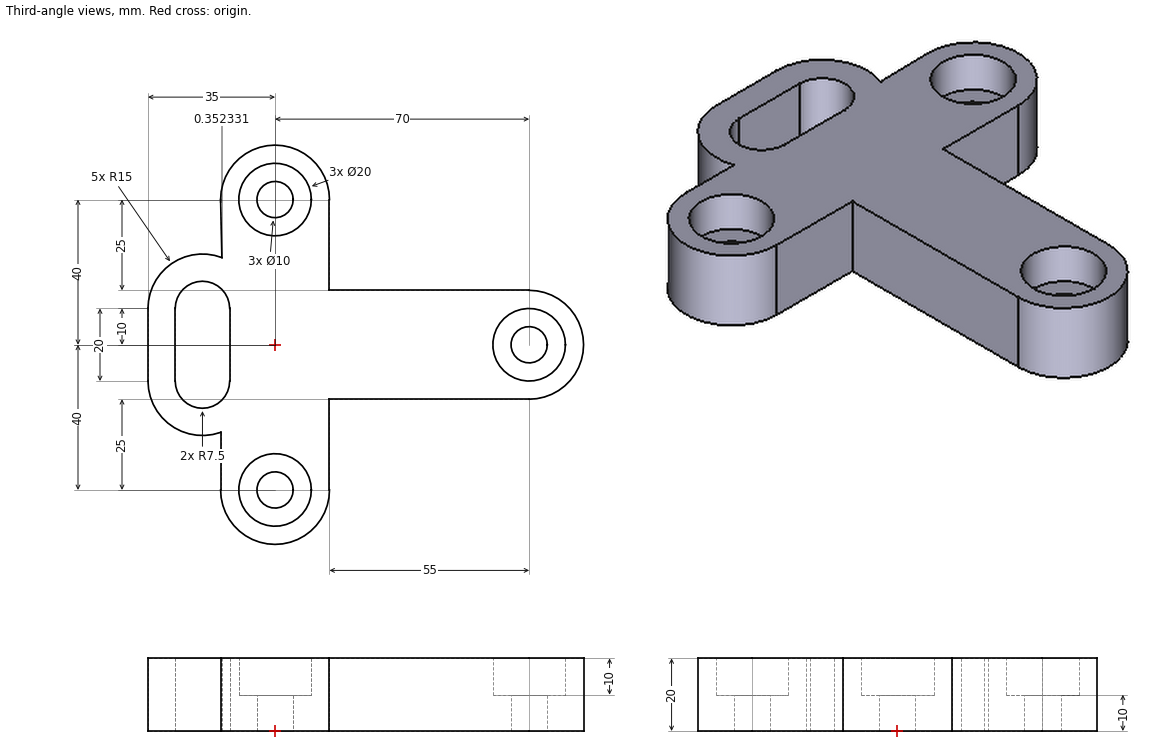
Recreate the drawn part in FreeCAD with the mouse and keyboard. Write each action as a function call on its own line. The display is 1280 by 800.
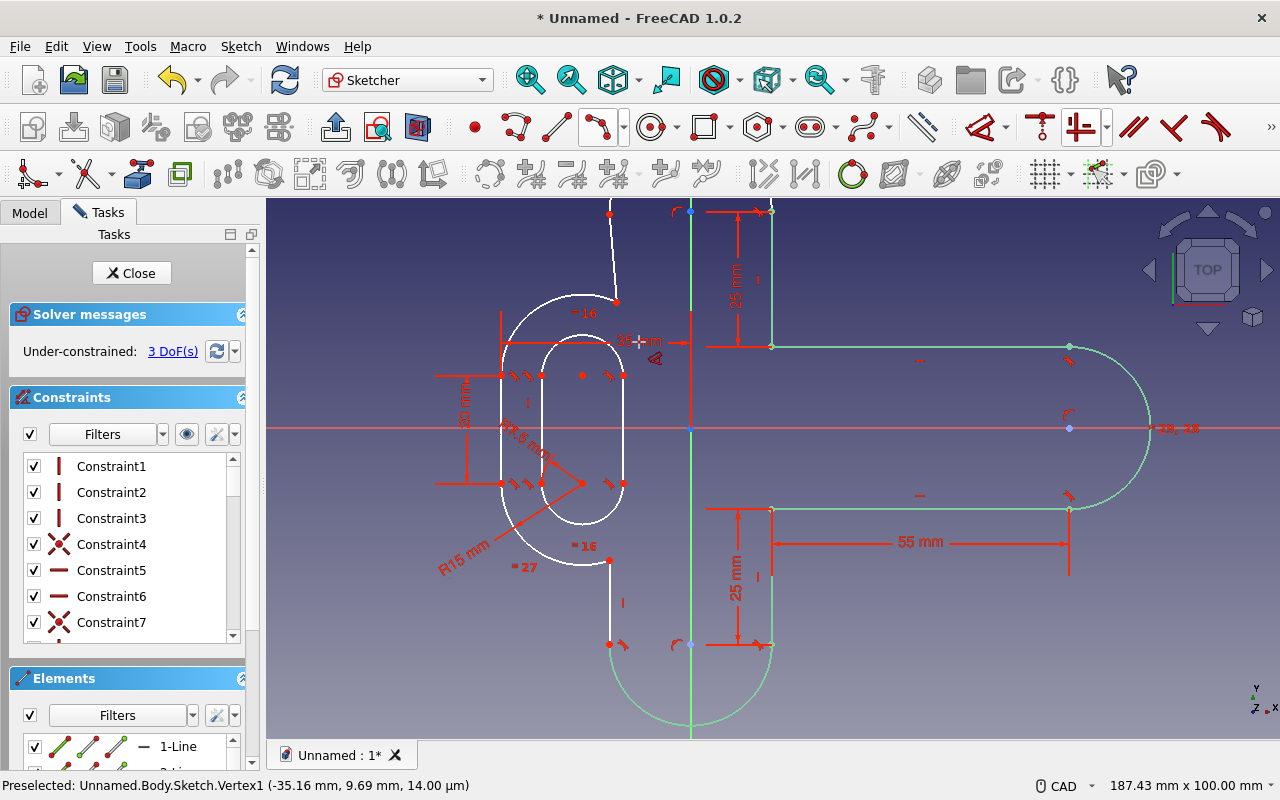
click(501, 376)
click(467, 384)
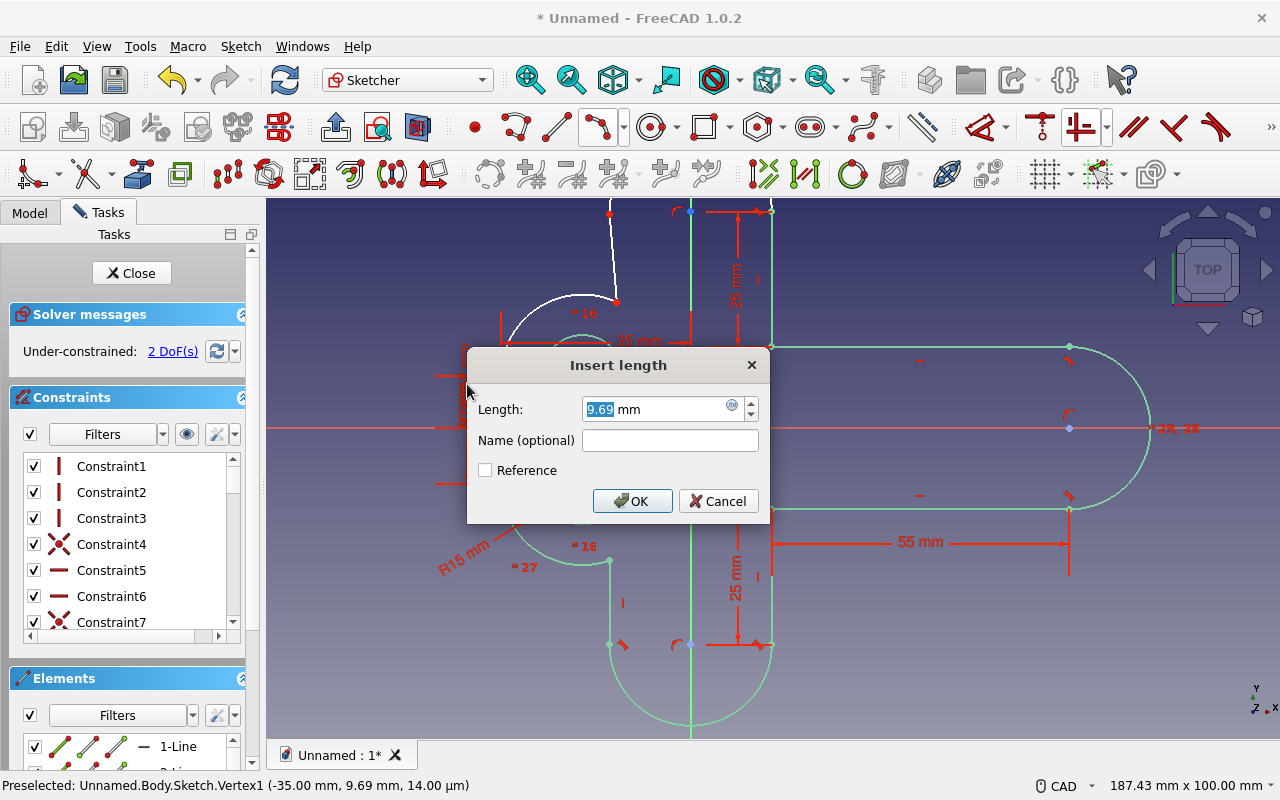
text(10)
key(Return)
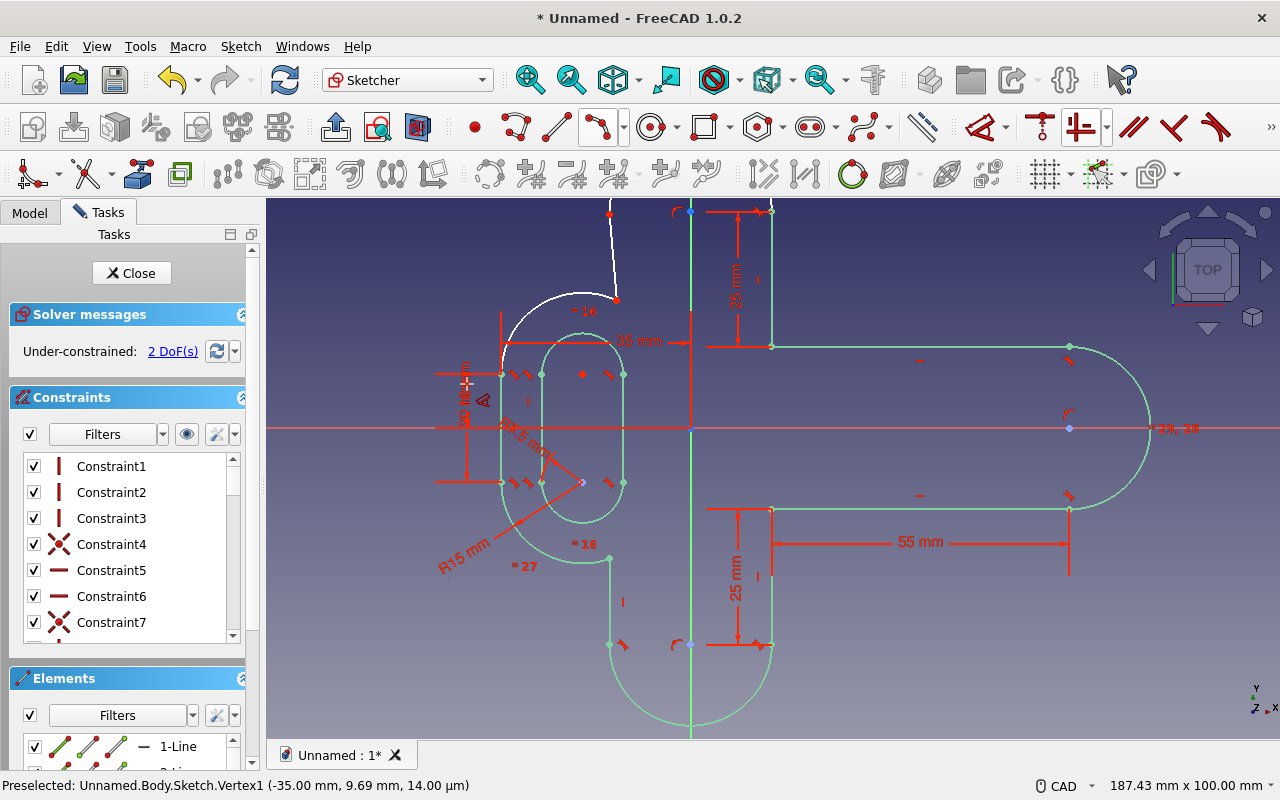
scroll(557, 518, down, 3)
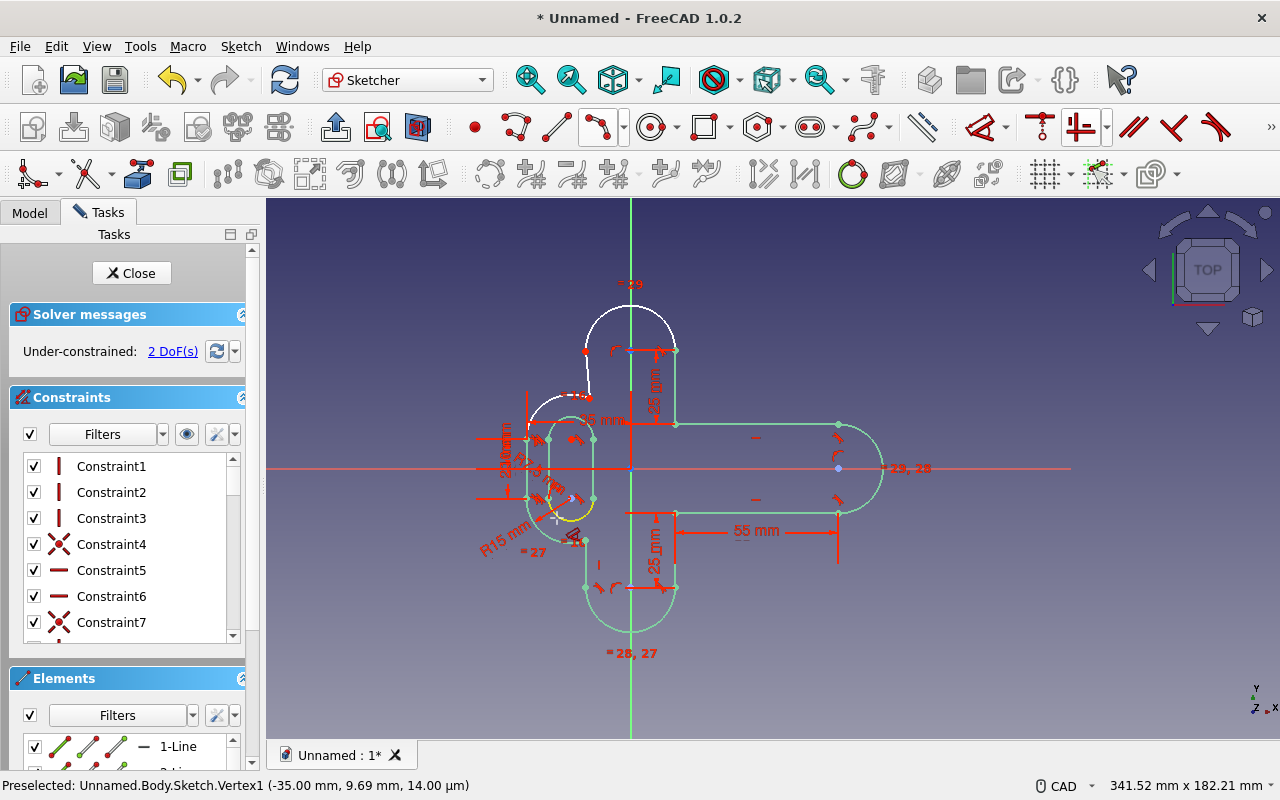
click(586, 351)
click(552, 383)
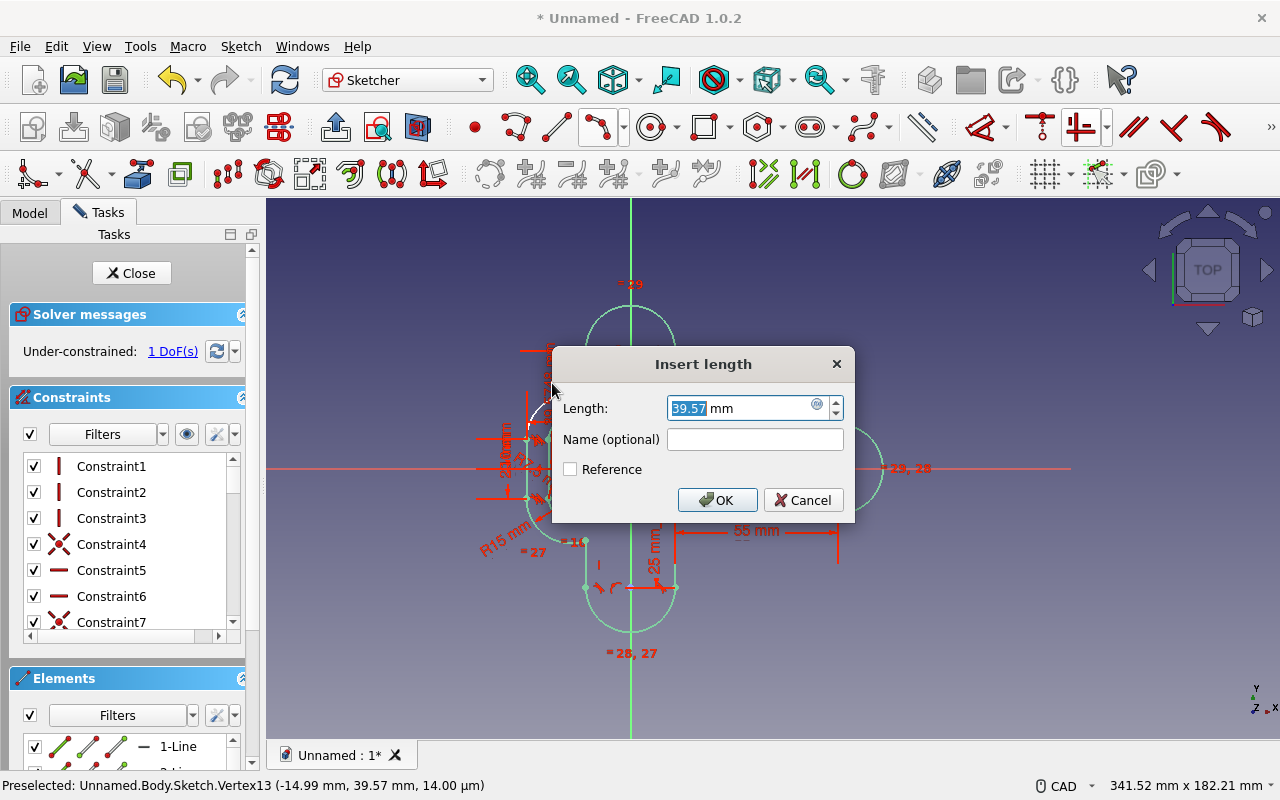
text(40)
key(Return)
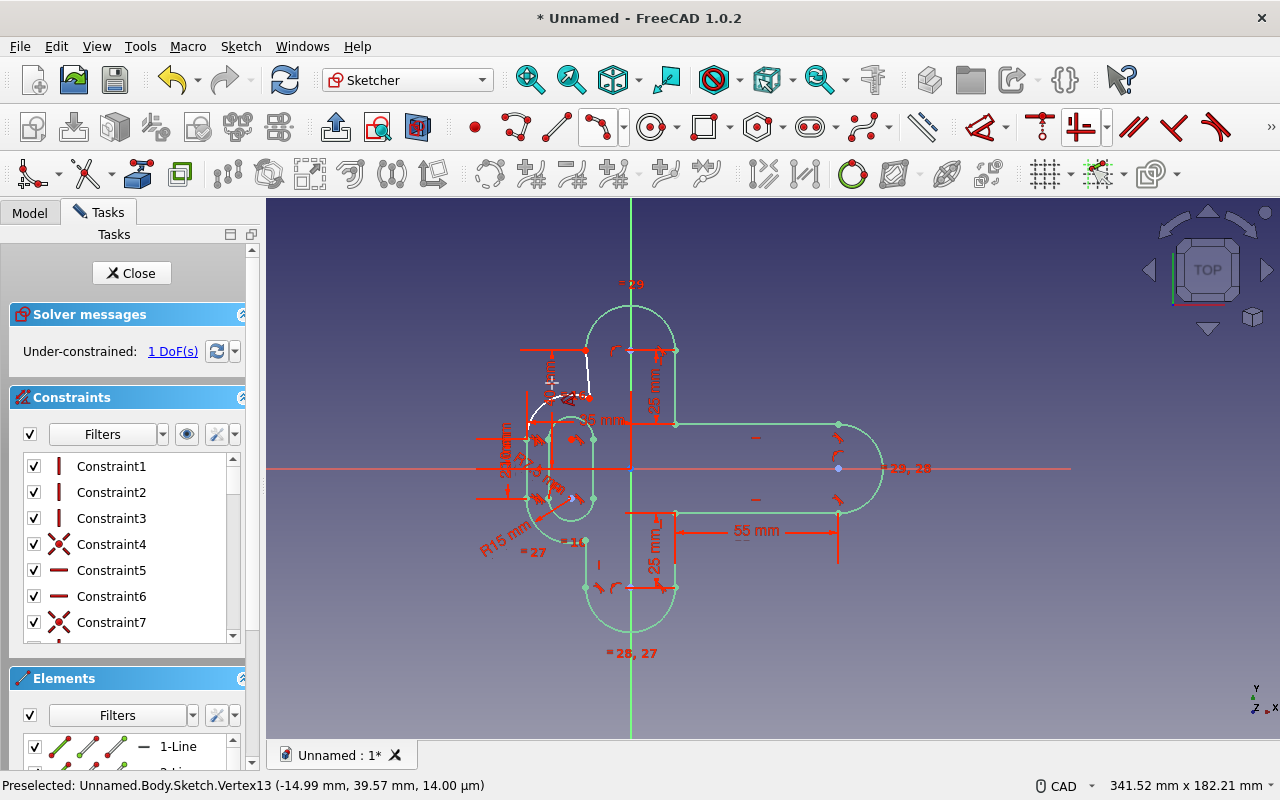
scroll(587, 365, up, 19)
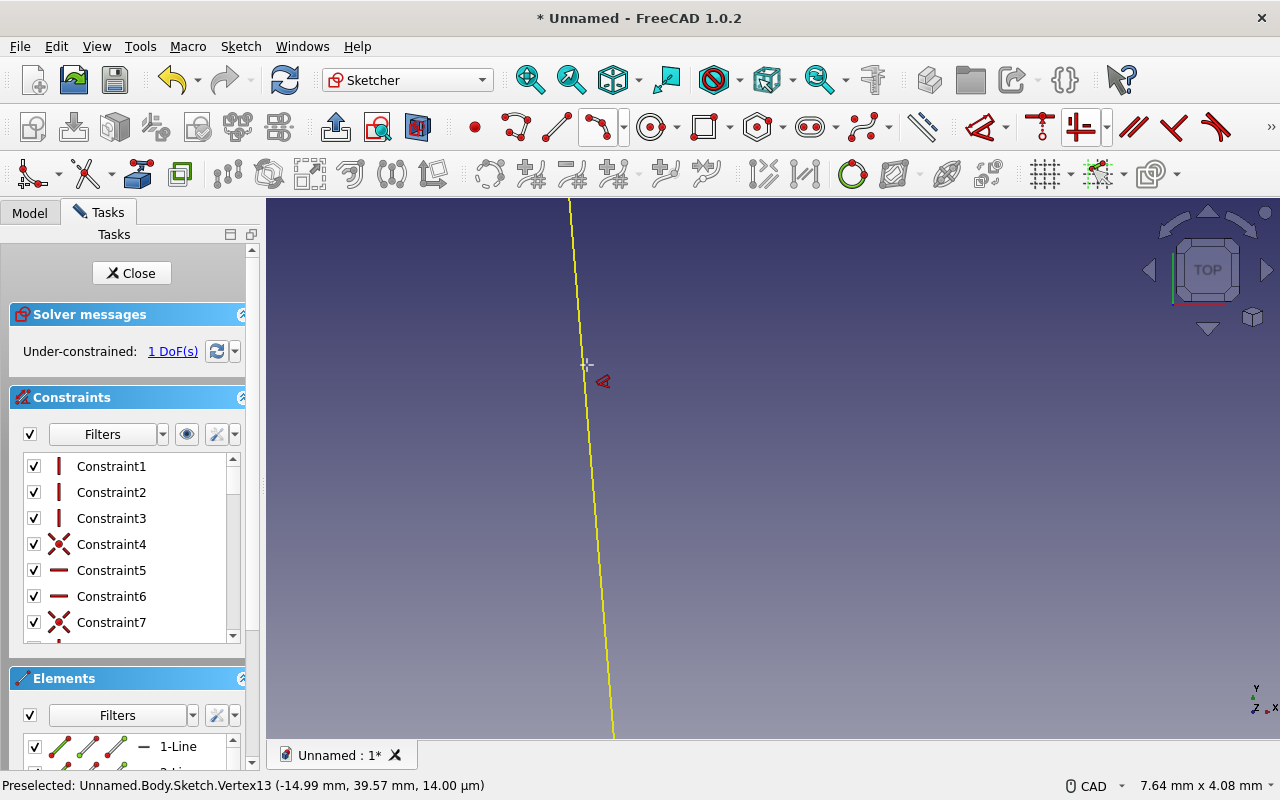
click(581, 343)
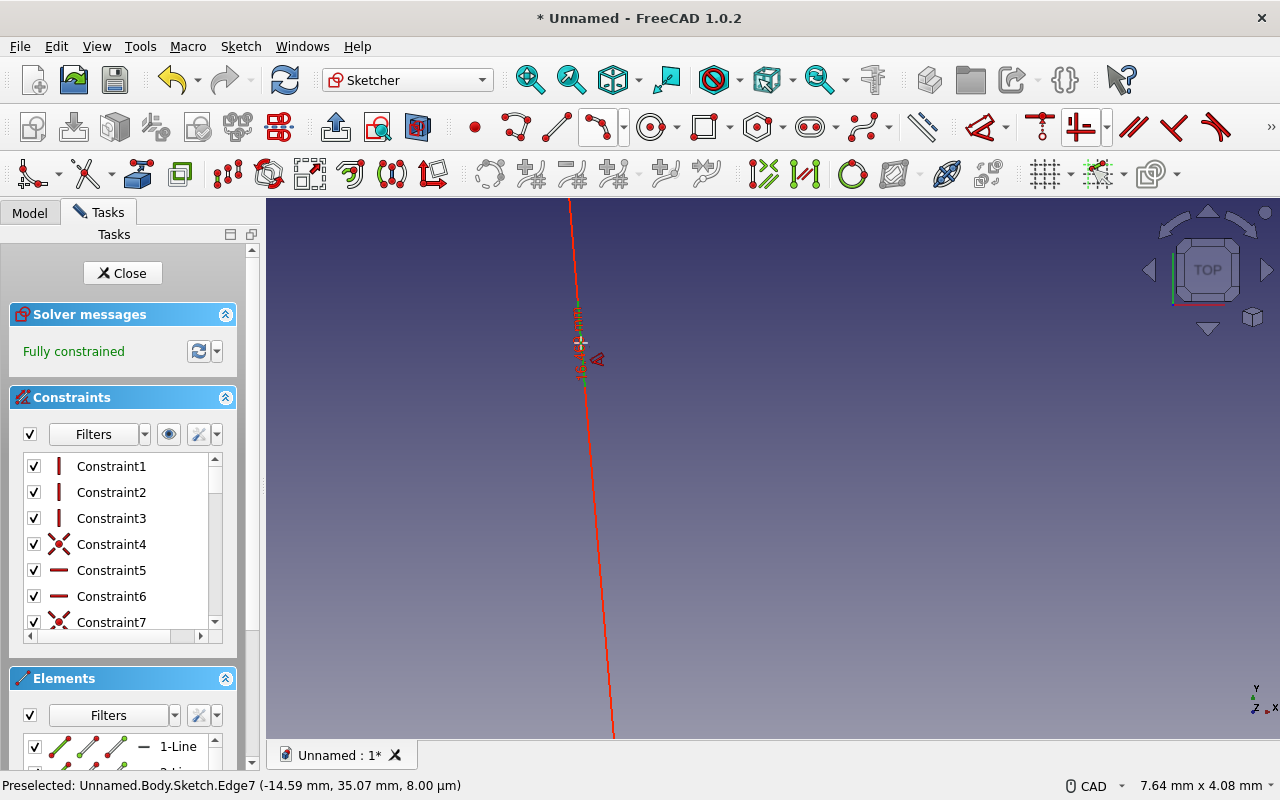
key(Escape)
key(Escape)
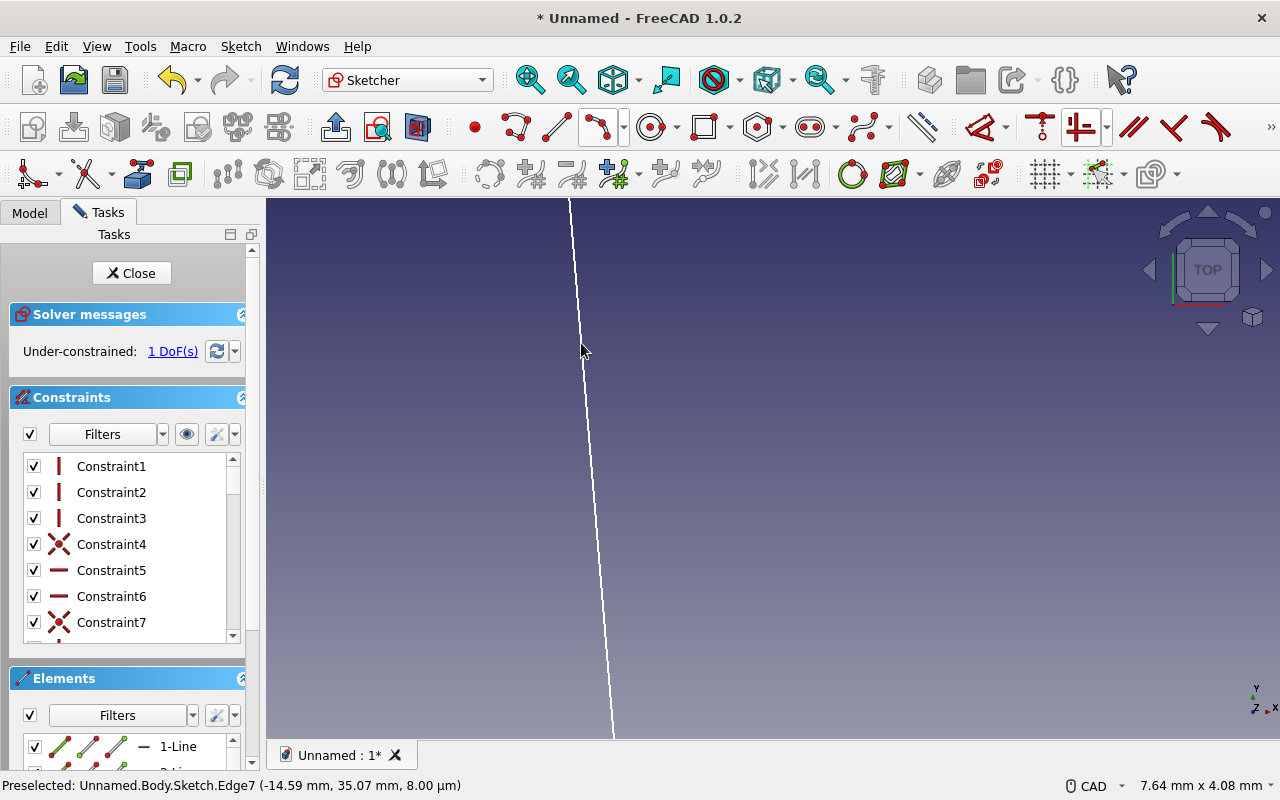
click(581, 343)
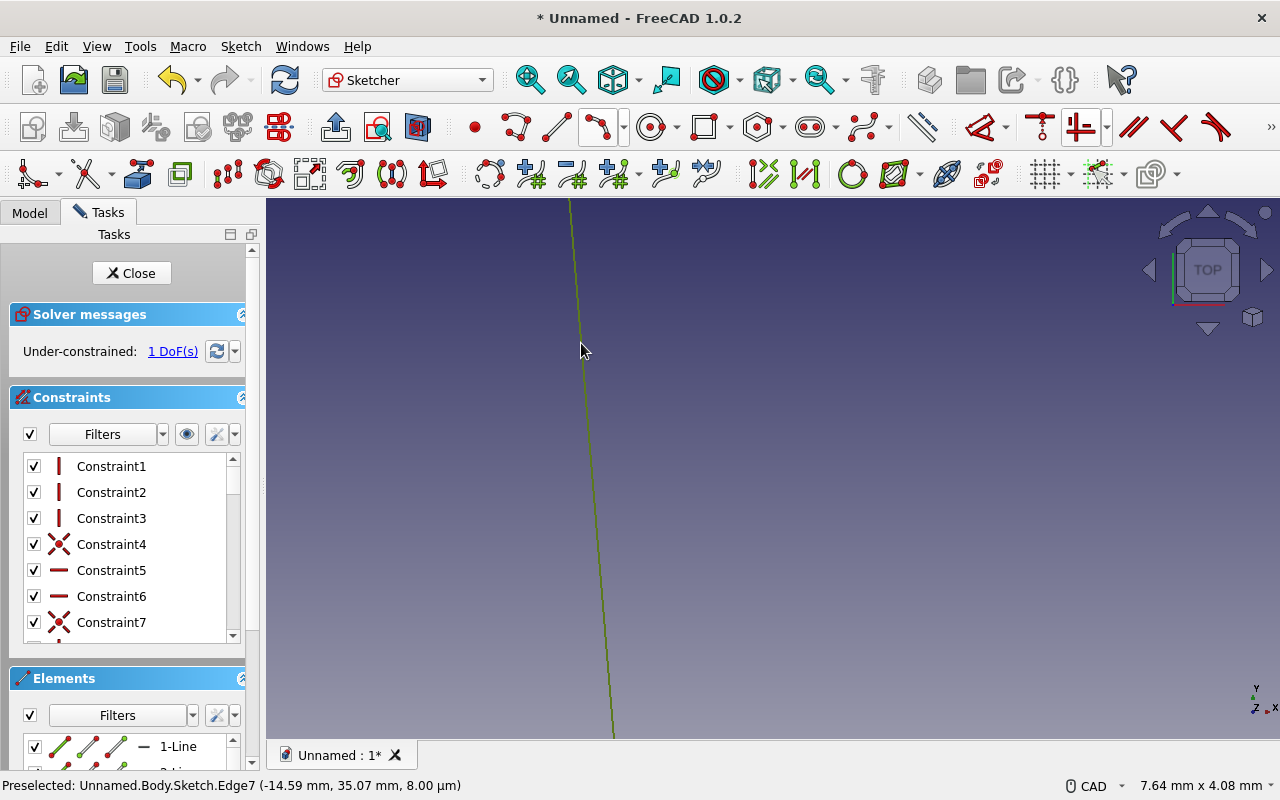
key(l)